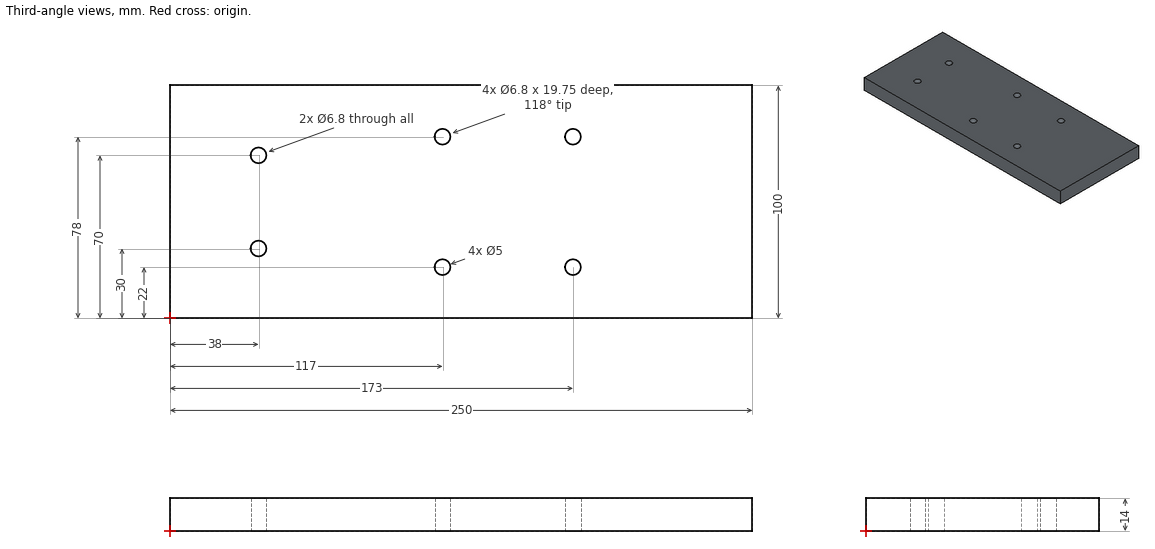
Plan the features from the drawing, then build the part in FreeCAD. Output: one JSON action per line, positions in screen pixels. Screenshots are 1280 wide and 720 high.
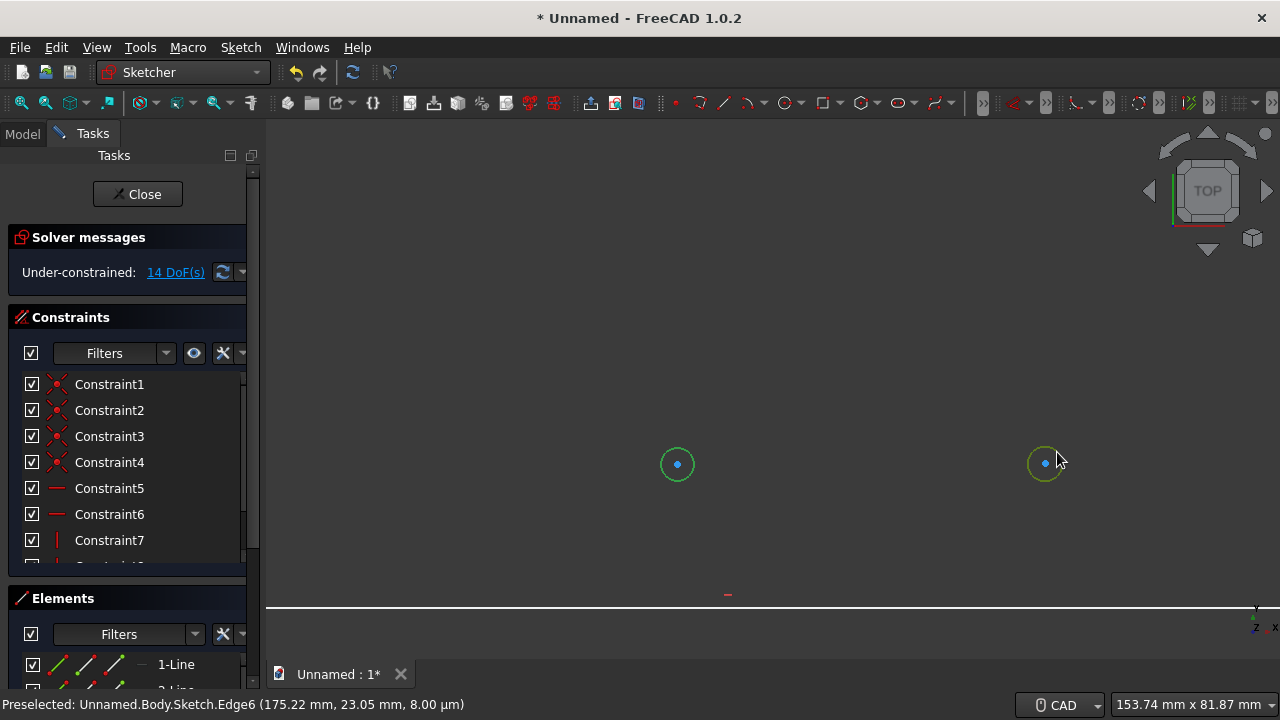
{"action": "scroll", "coordinate": [690, 454], "scroll_direction": "down", "scroll_amount": 5}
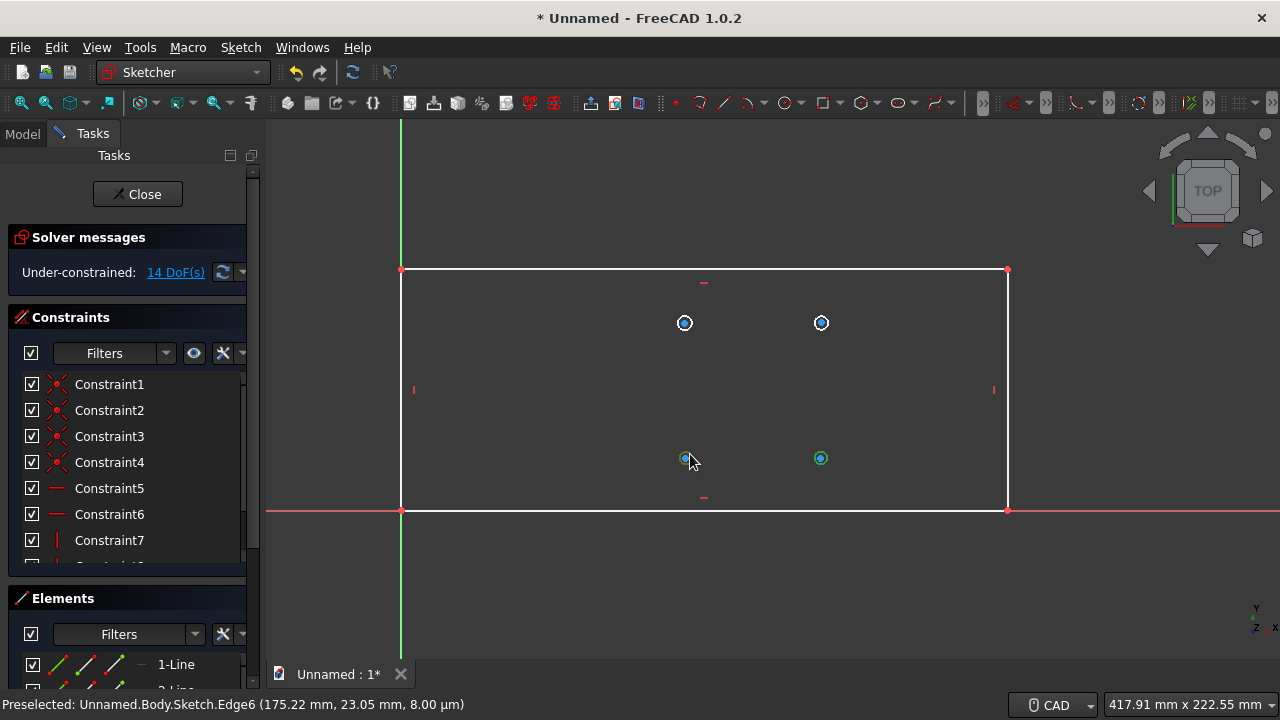
{"action": "scroll", "coordinate": [690, 318], "scroll_direction": "up", "scroll_amount": 4}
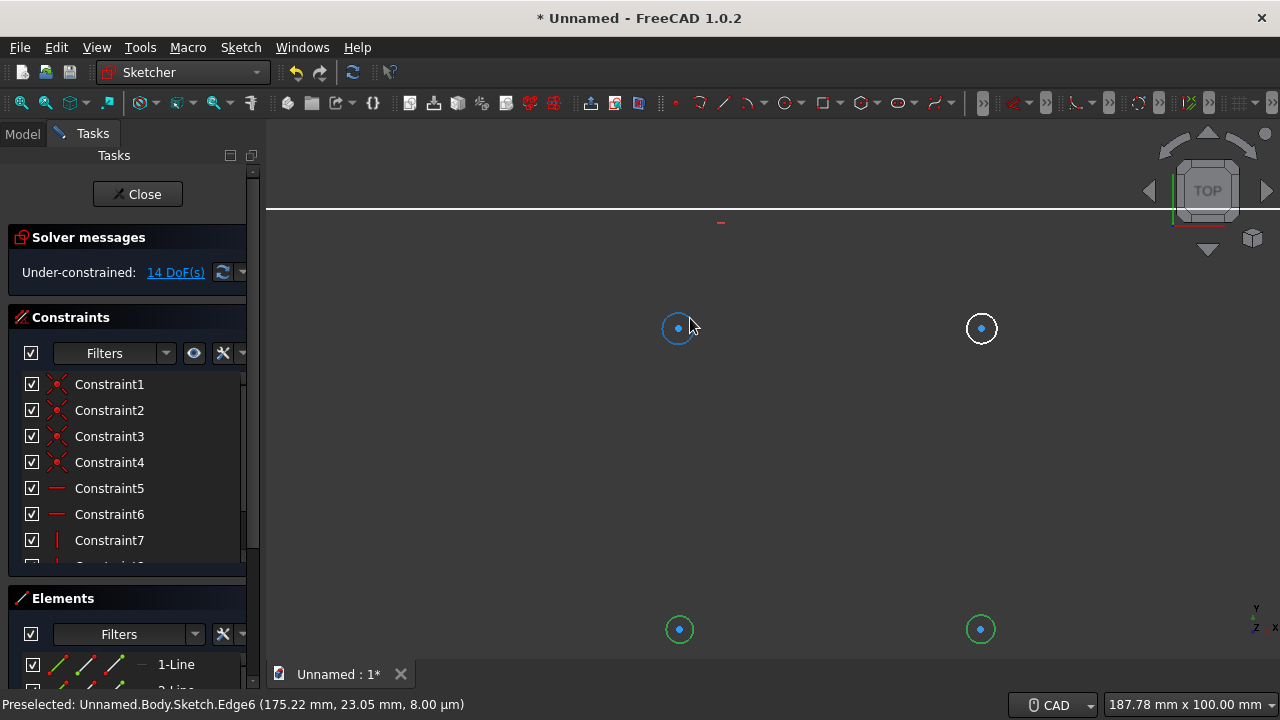
{"action": "left_click", "coordinate": [689, 318]}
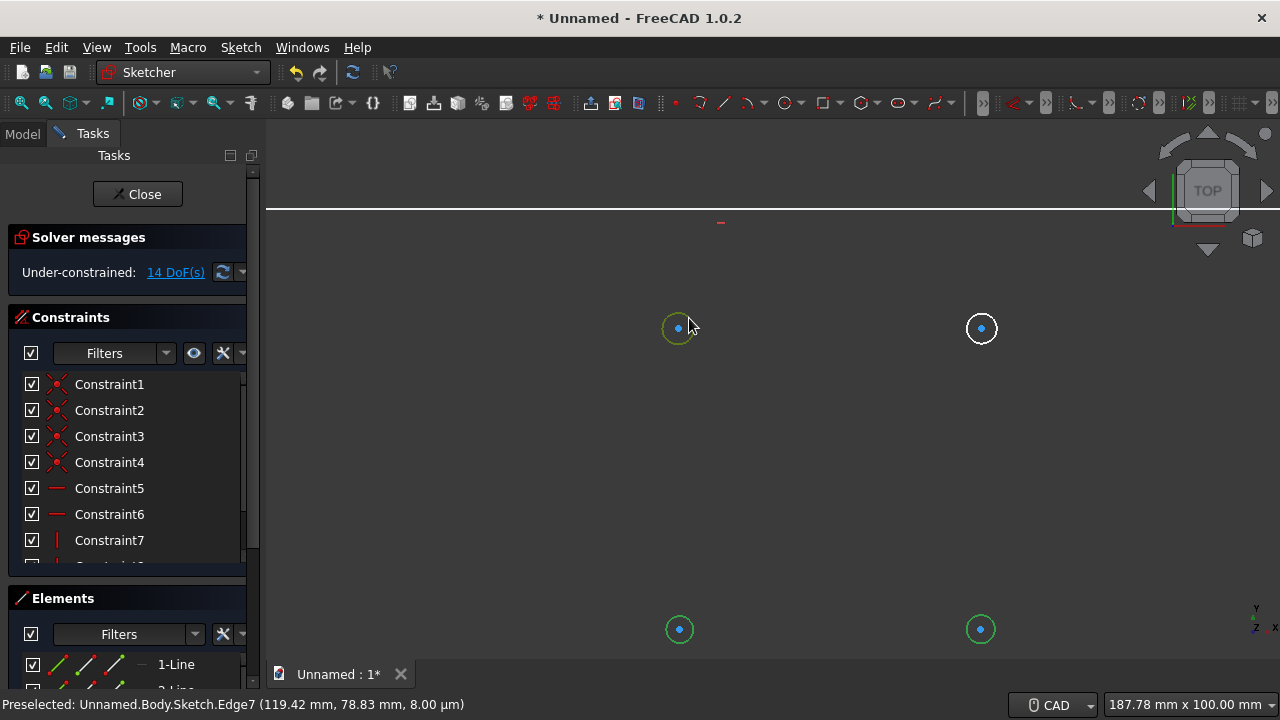
{"action": "left_click", "coordinate": [992, 318]}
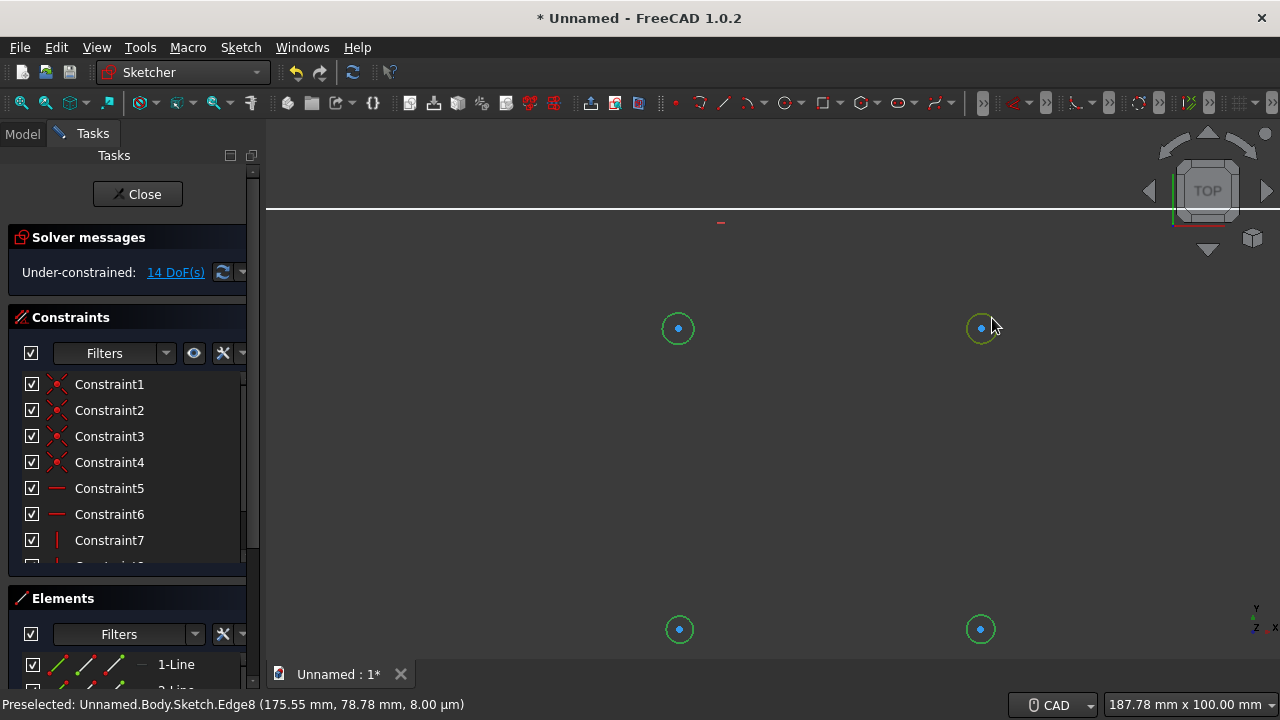
{"action": "key", "text": "e"}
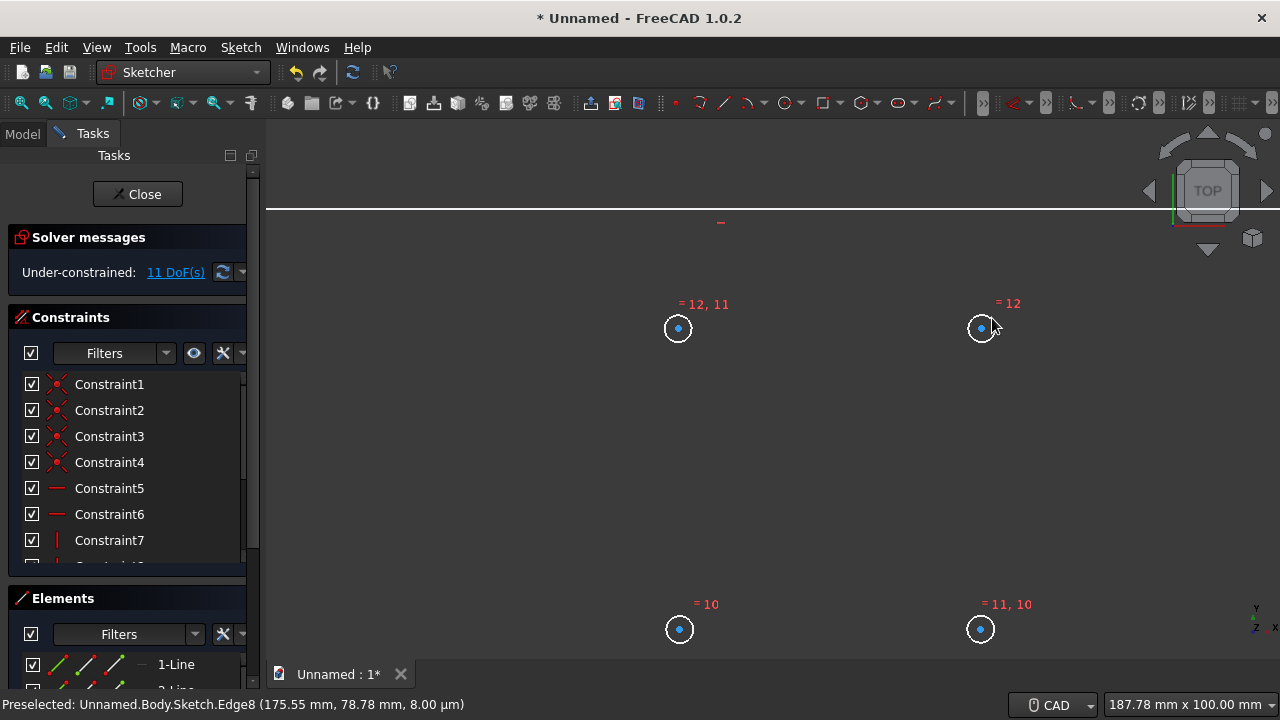
{"action": "left_click", "coordinate": [1014, 104]}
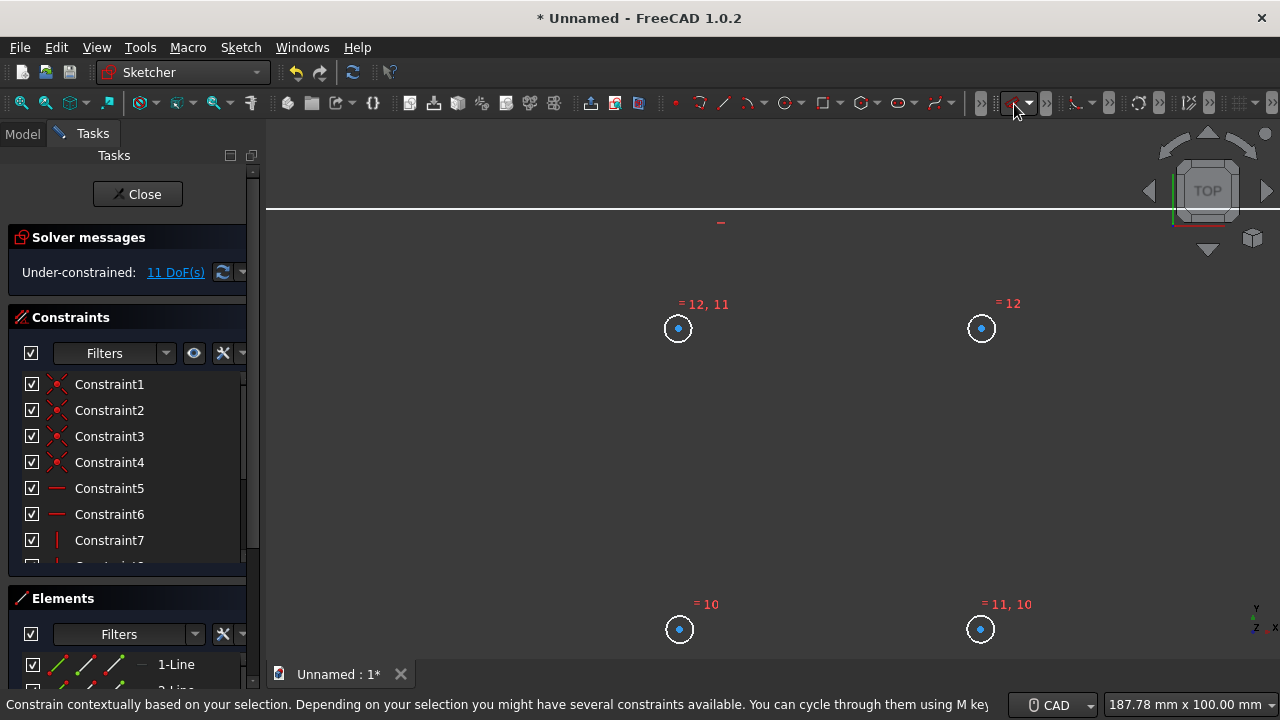
{"action": "scroll", "coordinate": [689, 620], "scroll_direction": "up", "scroll_amount": 2}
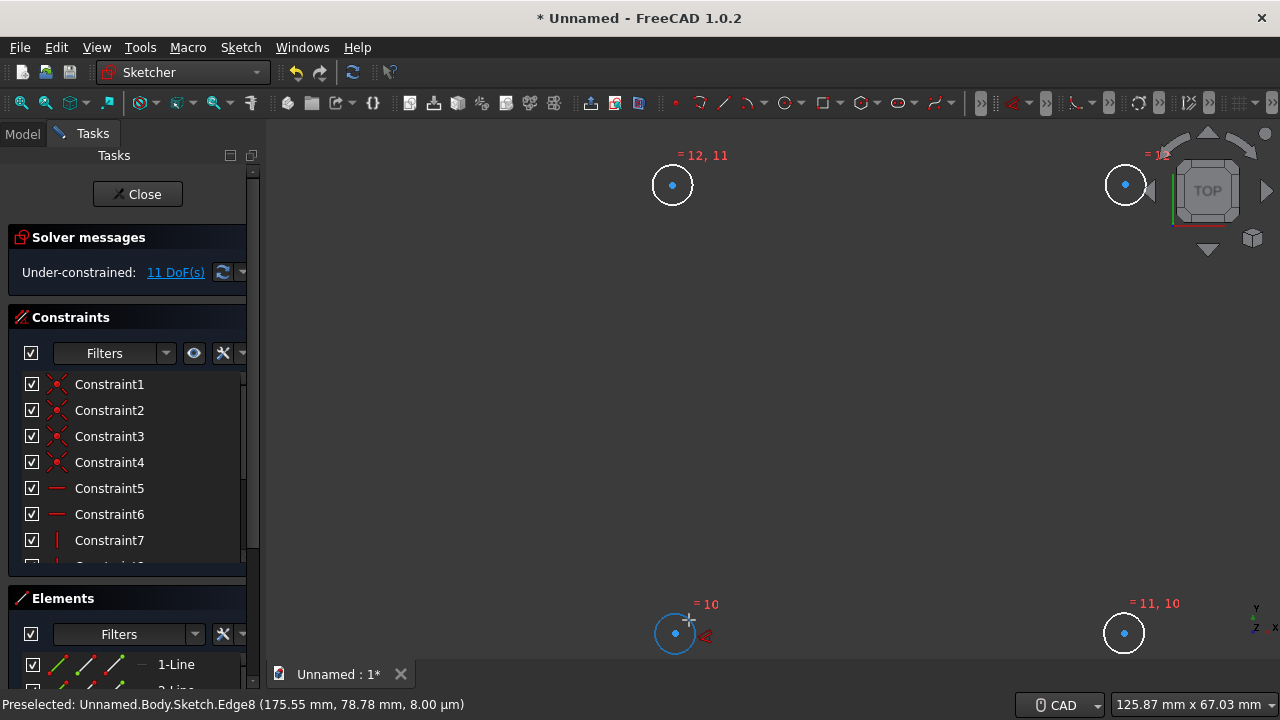
{"action": "left_click", "coordinate": [689, 620]}
{"action": "left_click", "coordinate": [712, 597]}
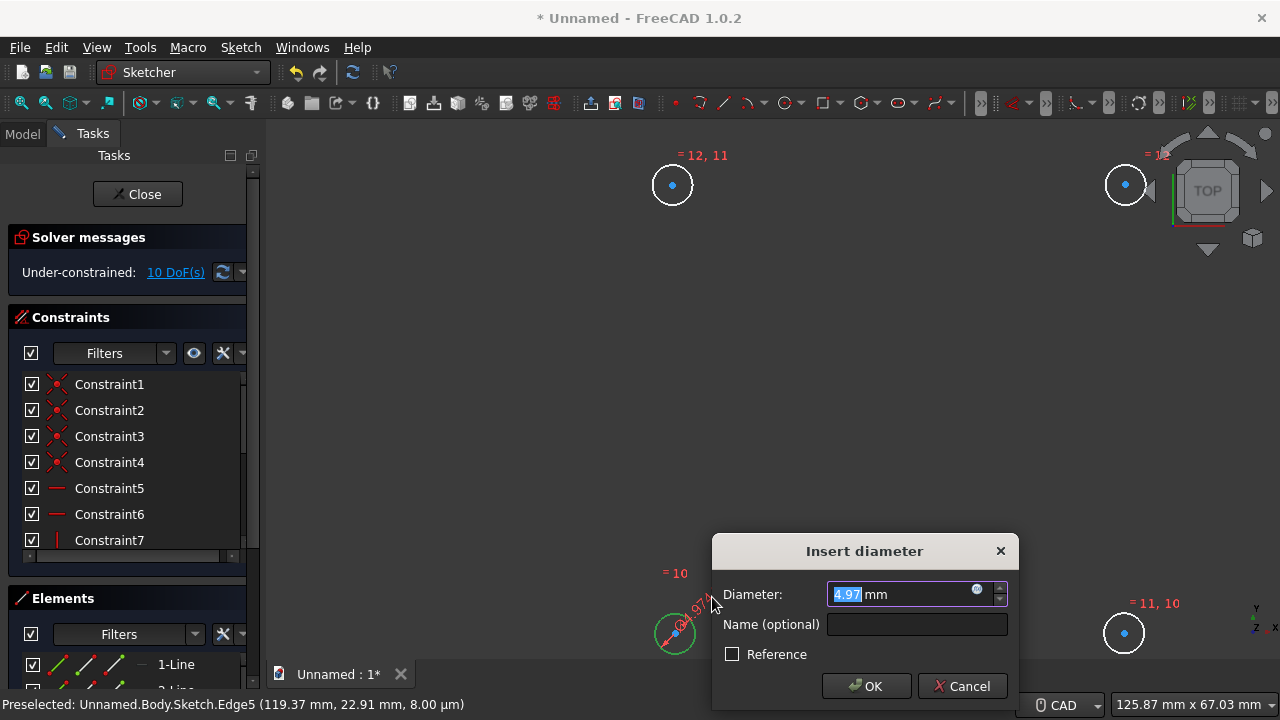
{"action": "type", "text": "5"}
{"action": "key", "text": "Return"}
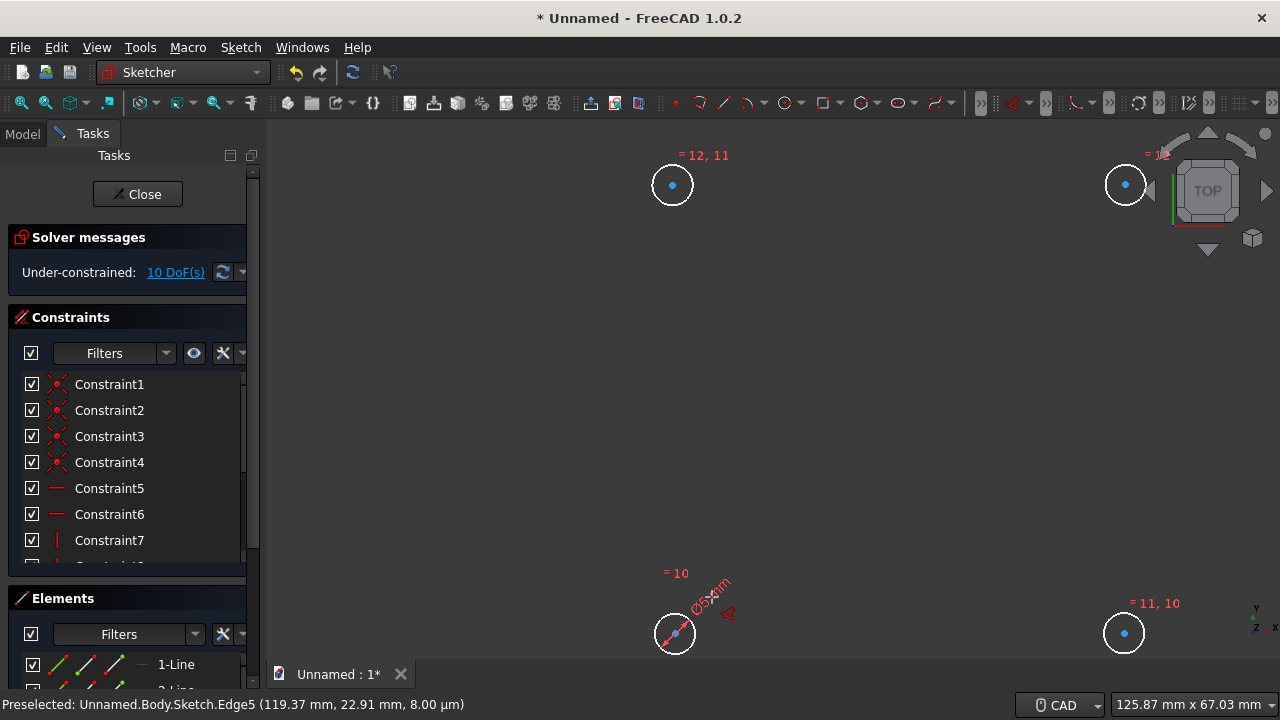
{"action": "scroll", "coordinate": [690, 382], "scroll_direction": "down", "scroll_amount": 6}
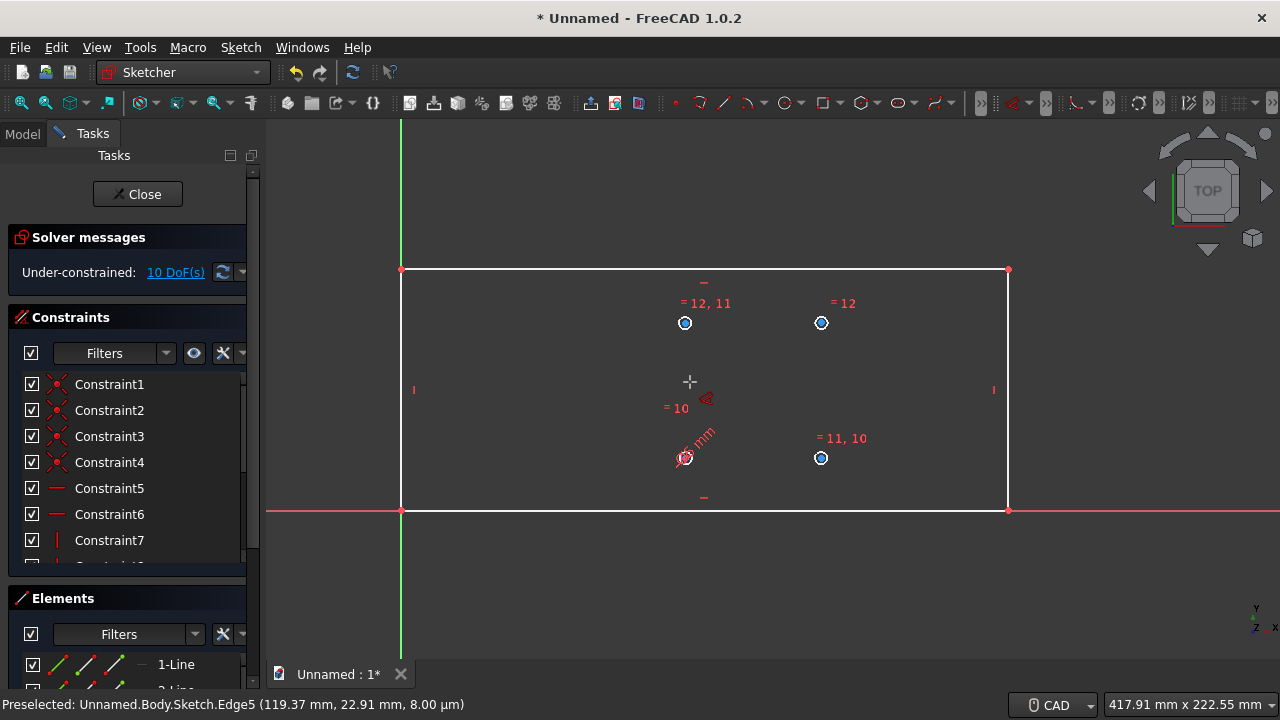
{"action": "left_click", "coordinate": [686, 458]}
{"action": "left_click", "coordinate": [367, 485]}